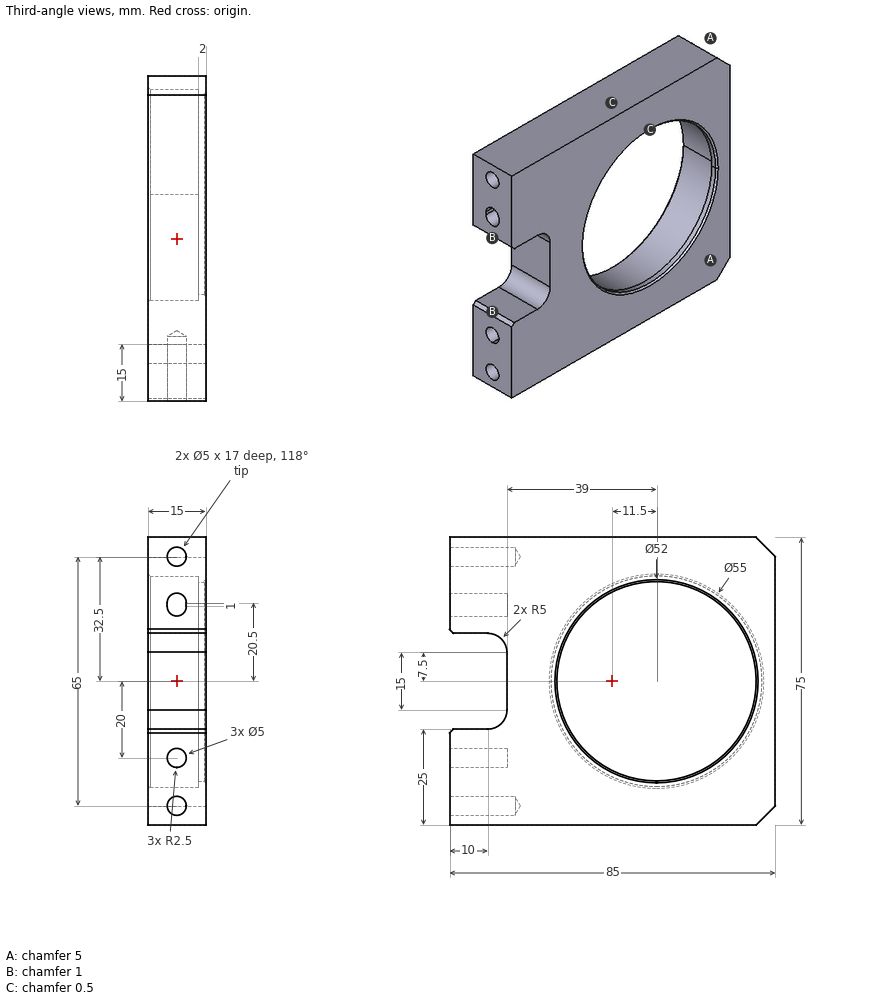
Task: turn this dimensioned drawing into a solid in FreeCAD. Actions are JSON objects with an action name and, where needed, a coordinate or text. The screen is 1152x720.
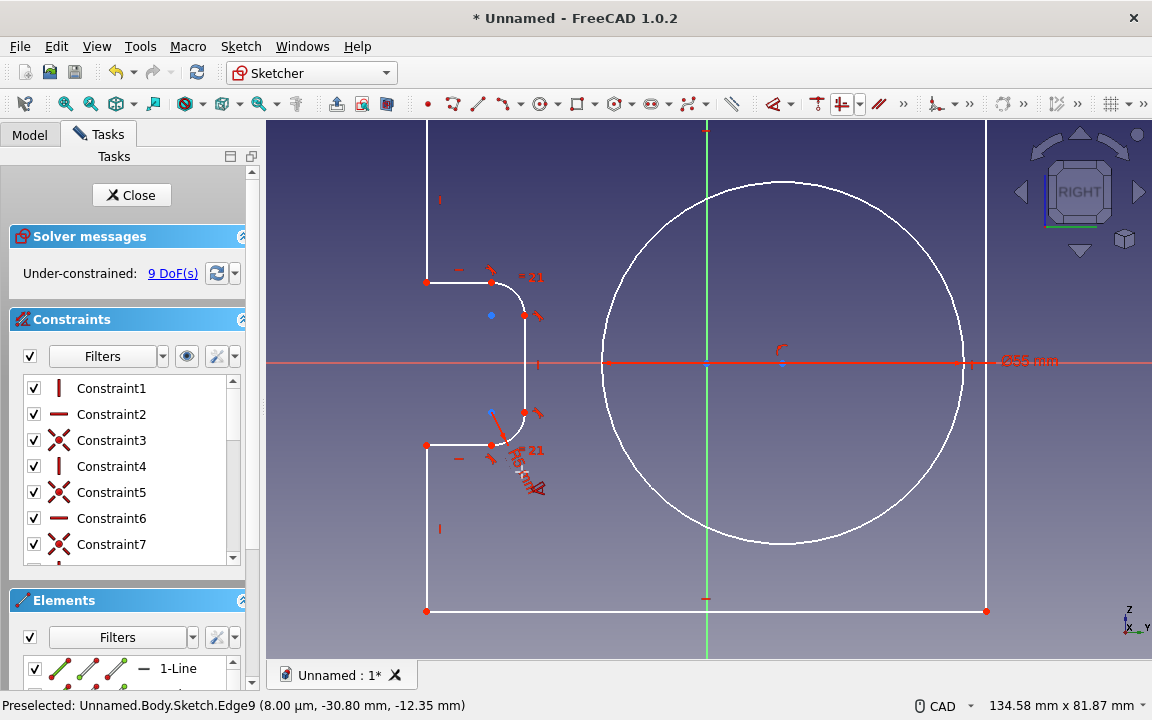
{"action": "left_click", "coordinate": [525, 345]}
{"action": "left_click", "coordinate": [491, 342]}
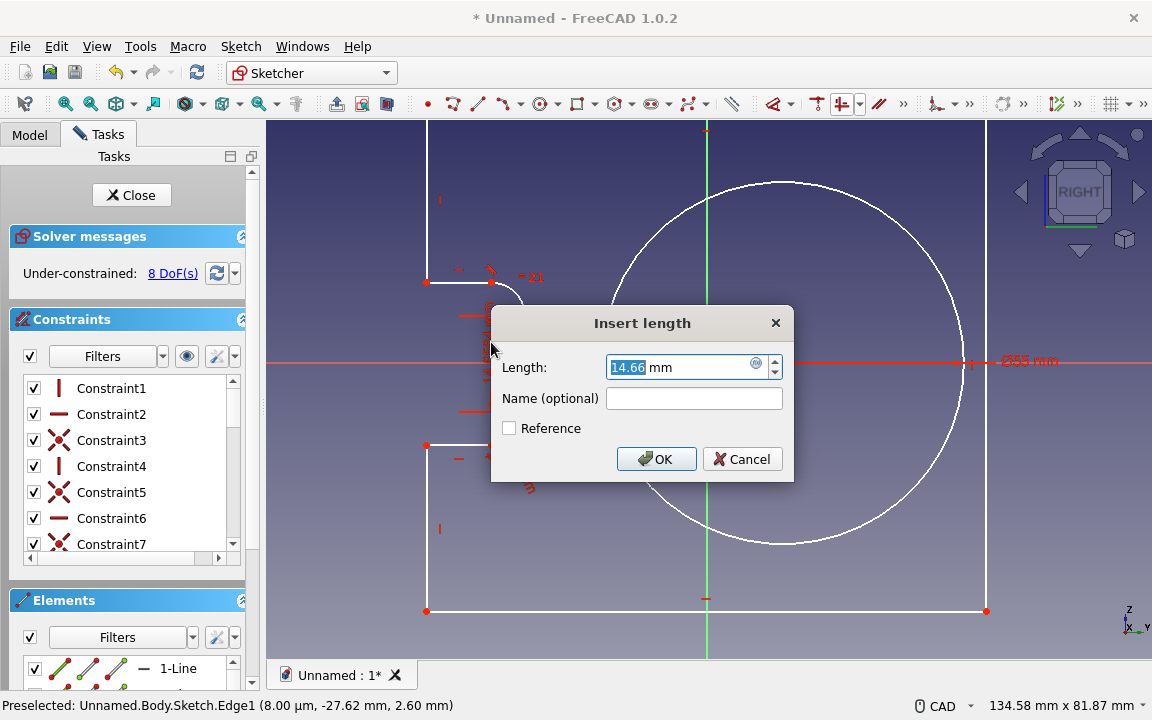
{"action": "type", "text": "15"}
{"action": "key", "text": "Return"}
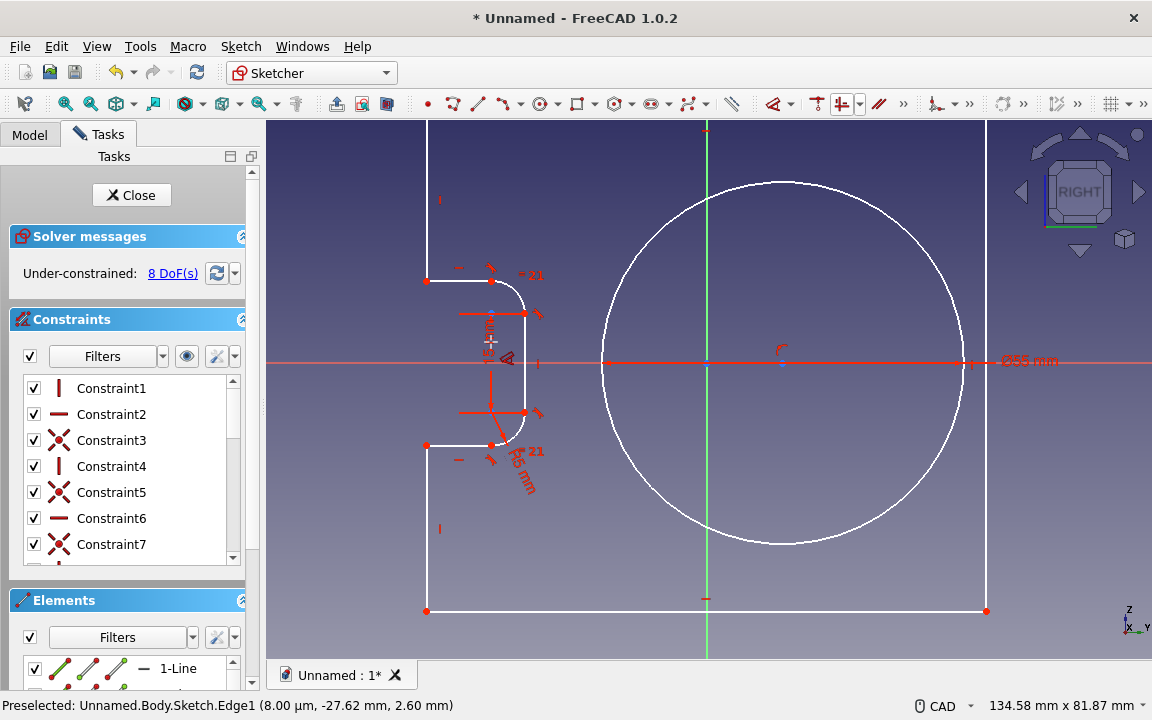
{"action": "left_click", "coordinate": [472, 446]}
{"action": "left_click", "coordinate": [444, 480]}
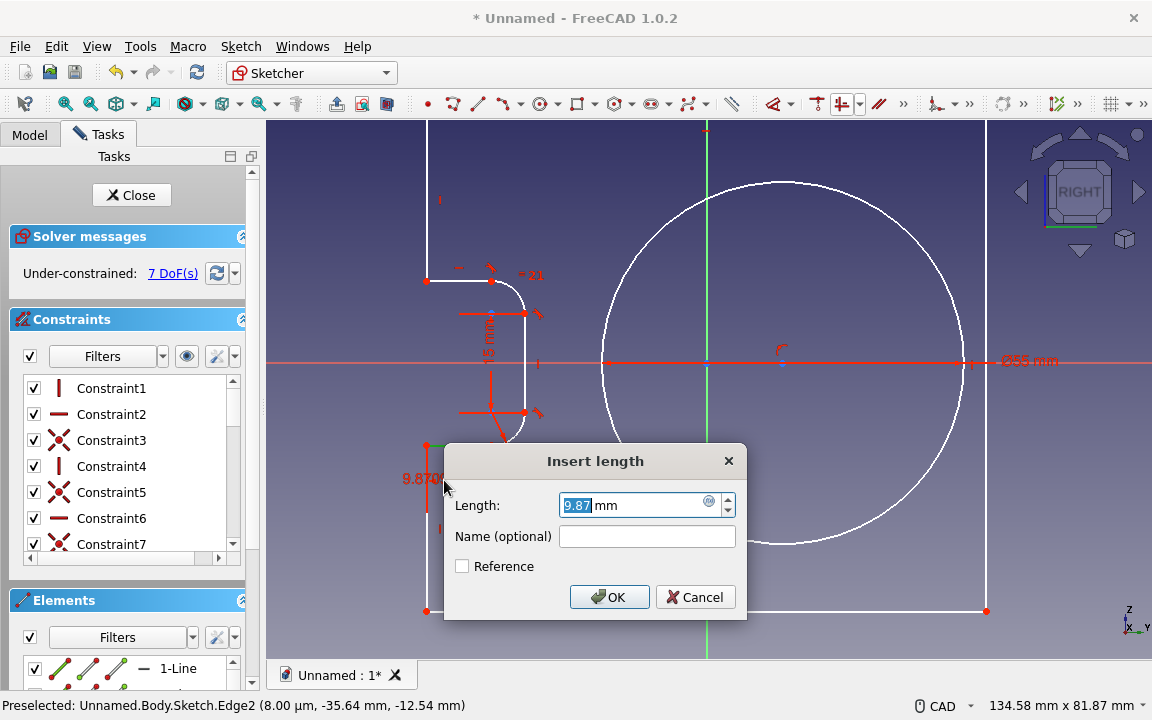
{"action": "type", "text": "10"}
{"action": "key", "text": "Return"}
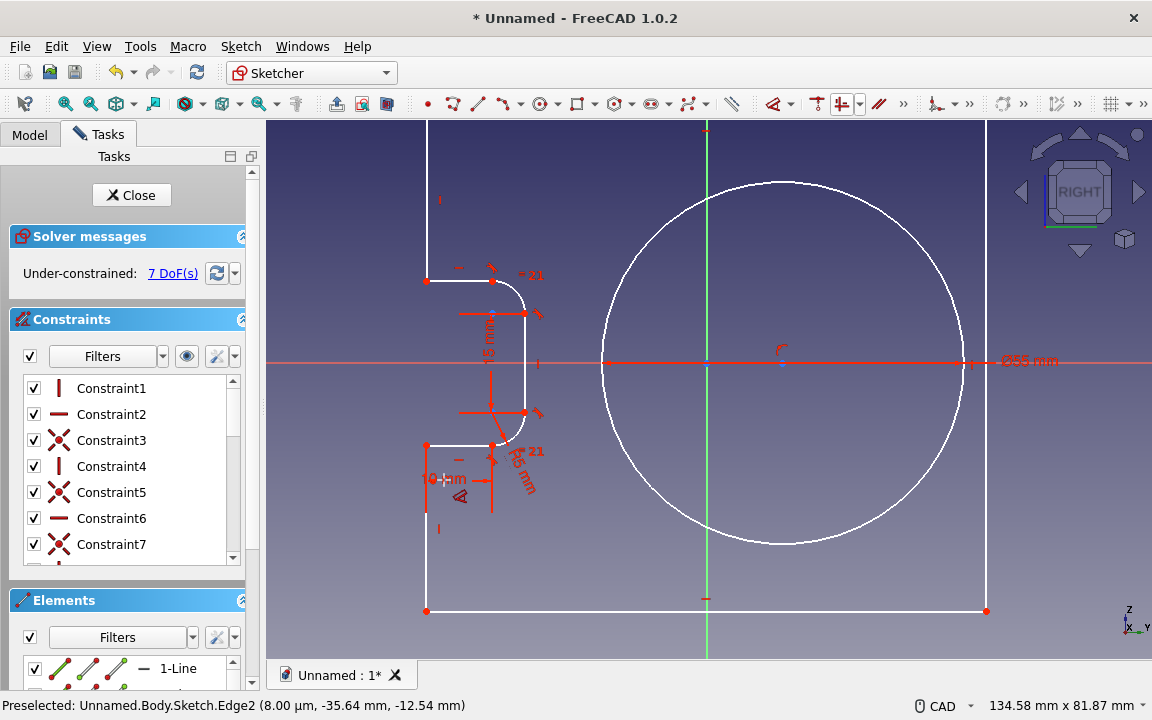
{"action": "left_click", "coordinate": [426, 495]}
{"action": "left_click", "coordinate": [392, 529]}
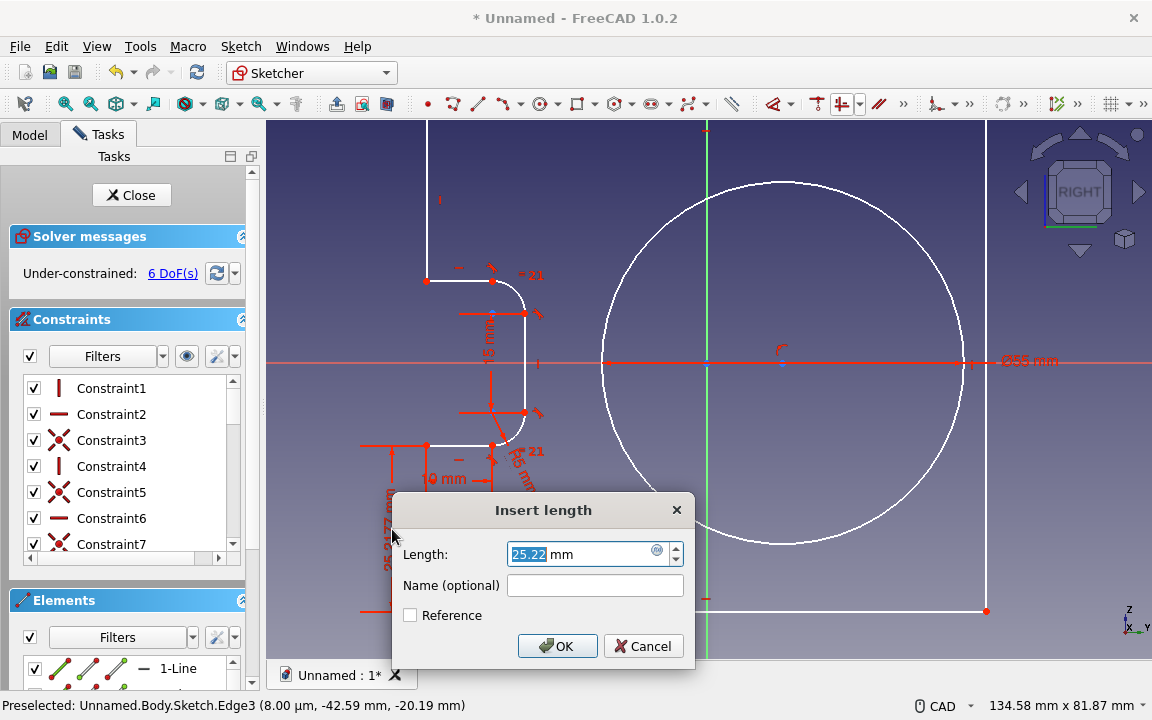
{"action": "type", "text": "25"}
{"action": "key", "text": "Return"}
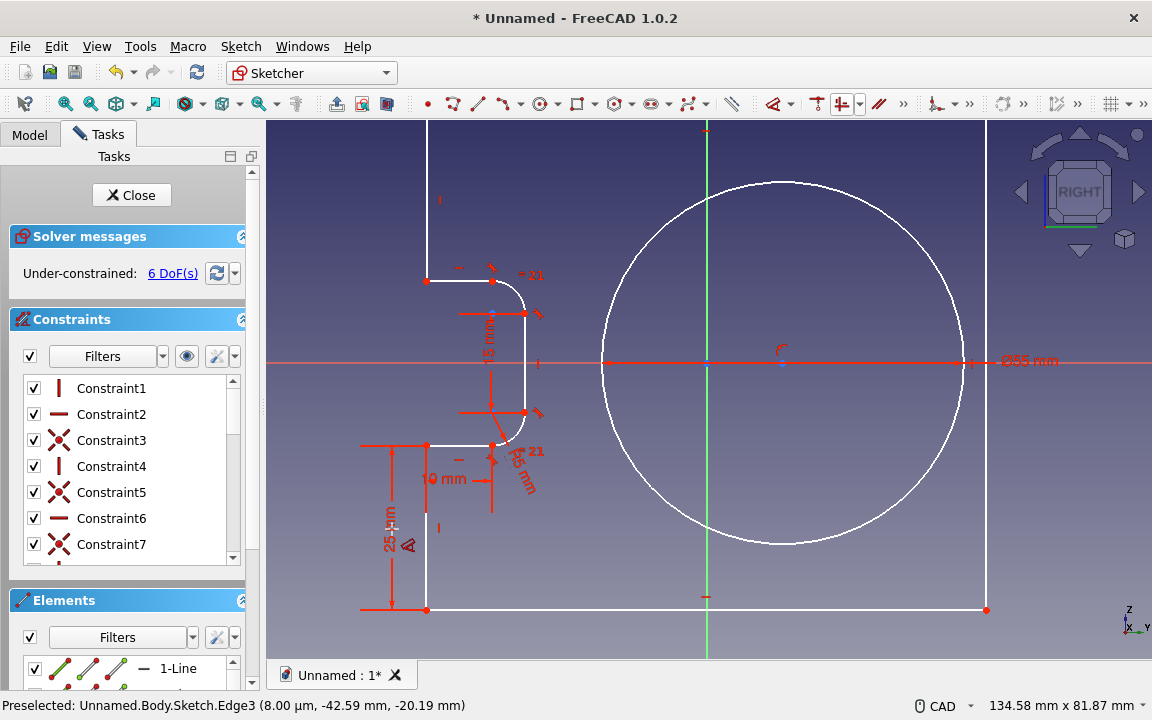
{"action": "left_click", "coordinate": [594, 610]}
{"action": "left_click", "coordinate": [577, 576]}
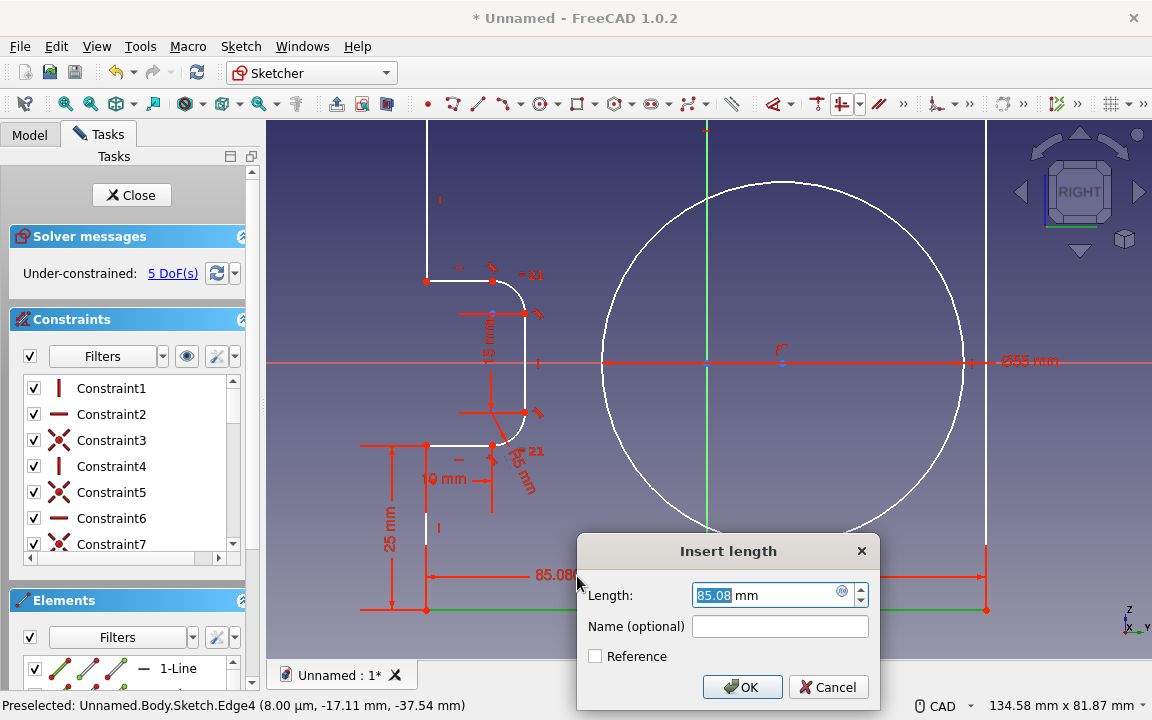
{"action": "type", "text": "85"}
{"action": "key", "text": "Return"}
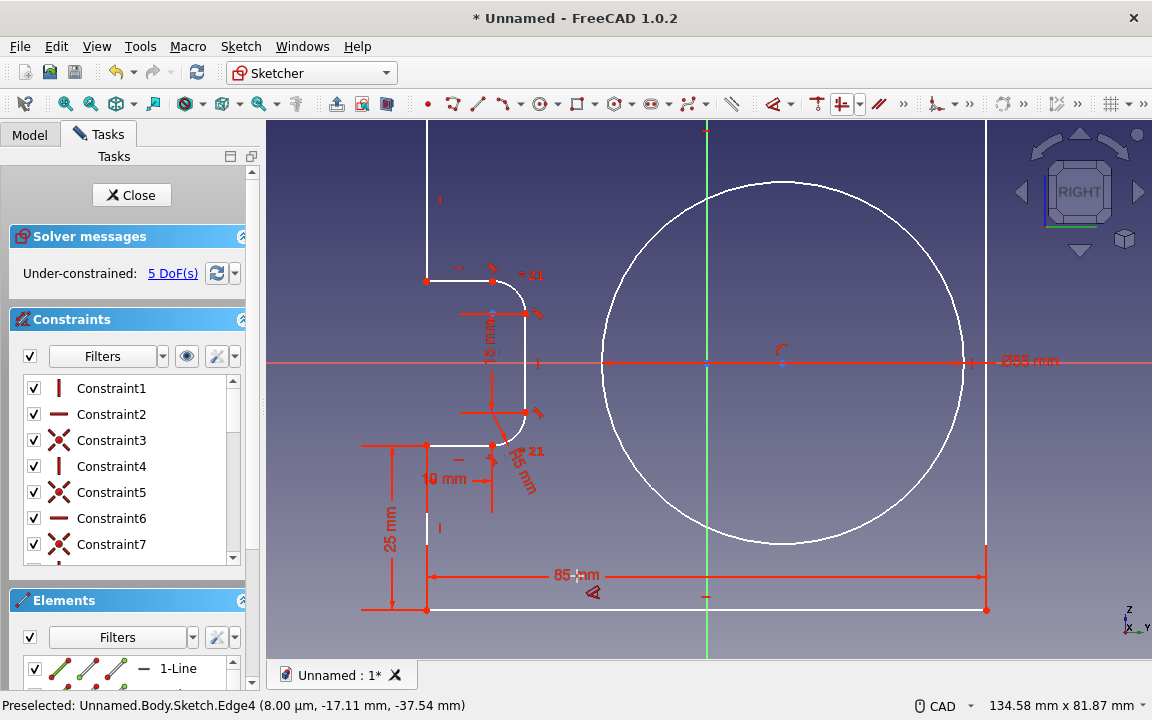
{"action": "left_click", "coordinate": [986, 462]}
{"action": "left_click", "coordinate": [952, 485]}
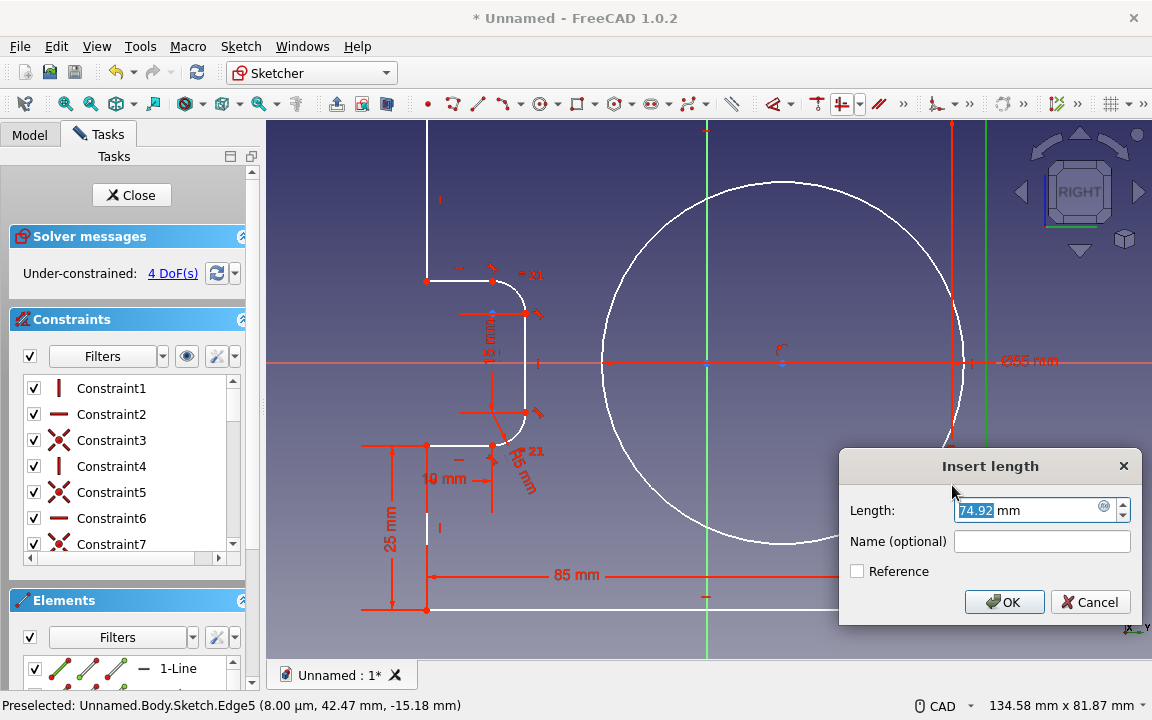
{"action": "type", "text": "75"}
{"action": "key", "text": "Return"}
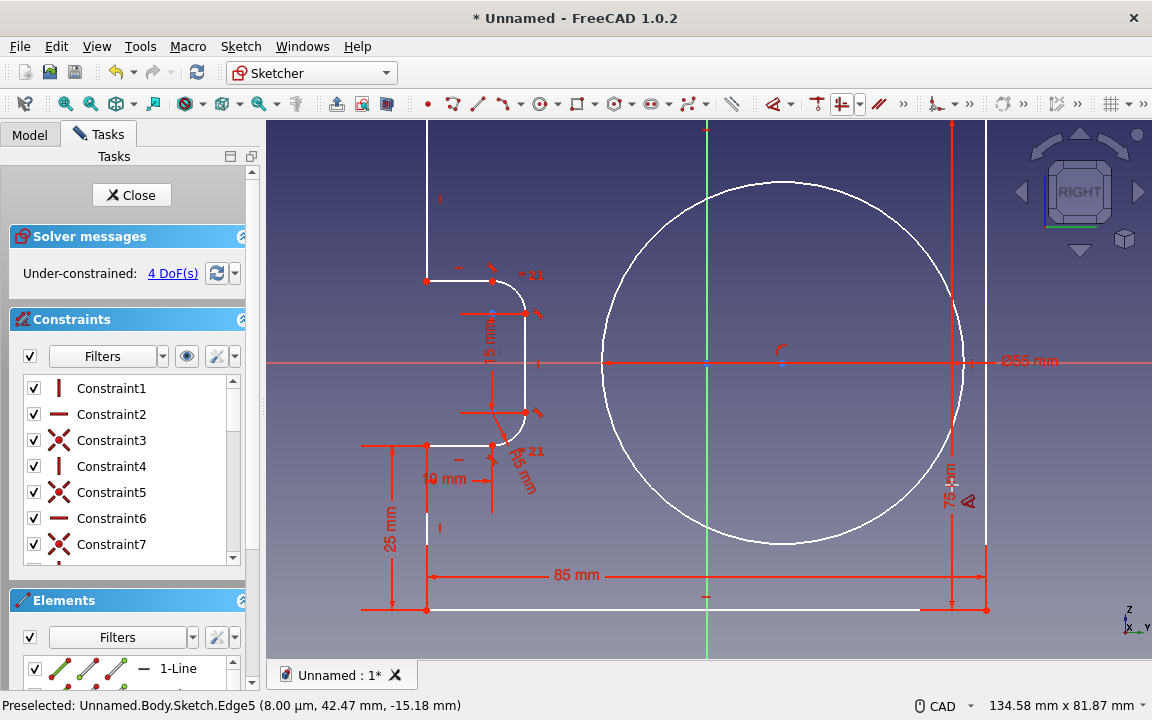
{"action": "scroll", "coordinate": [506, 443], "scroll_direction": "down", "scroll_amount": 2}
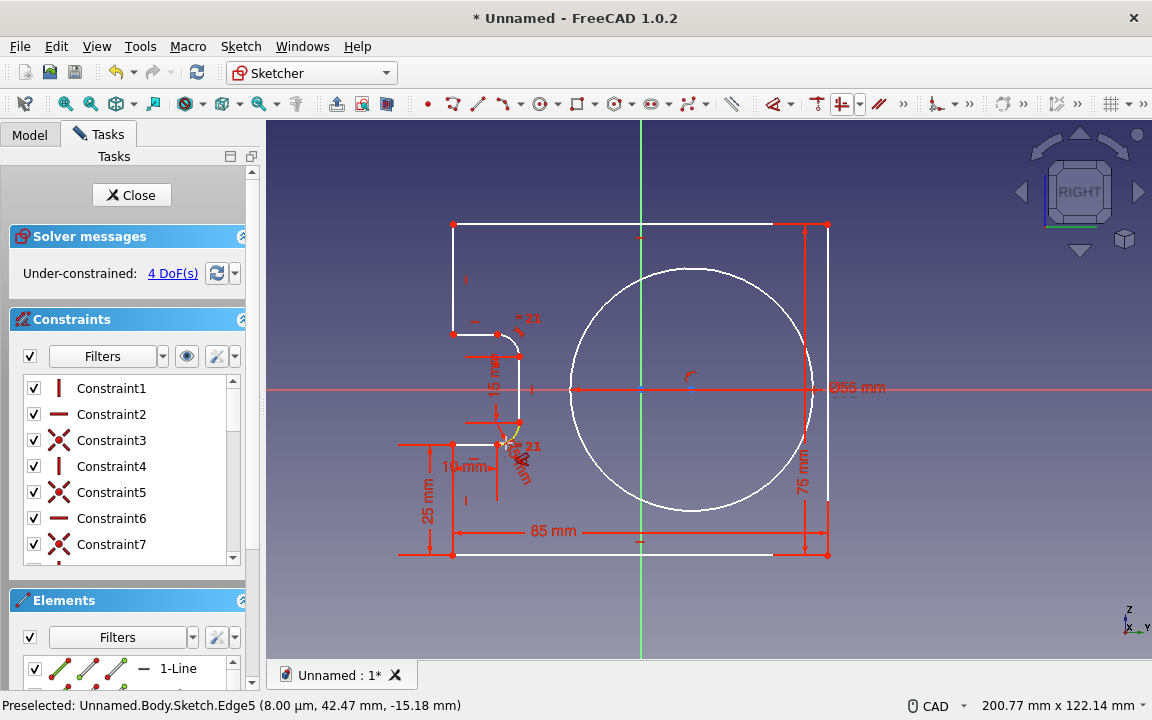
{"action": "left_click", "coordinate": [716, 224]}
{"action": "left_click", "coordinate": [554, 190]}